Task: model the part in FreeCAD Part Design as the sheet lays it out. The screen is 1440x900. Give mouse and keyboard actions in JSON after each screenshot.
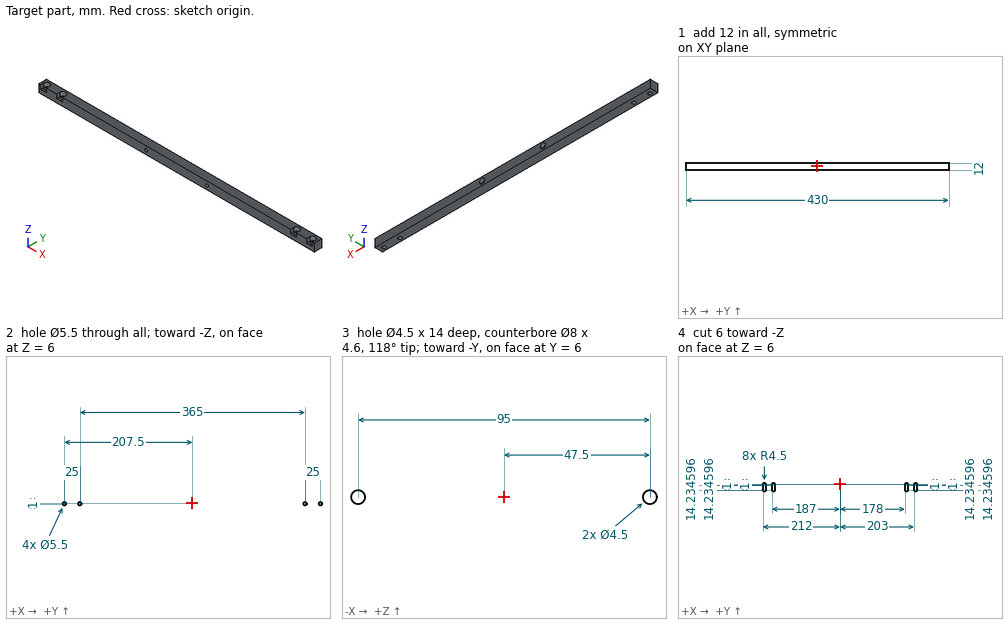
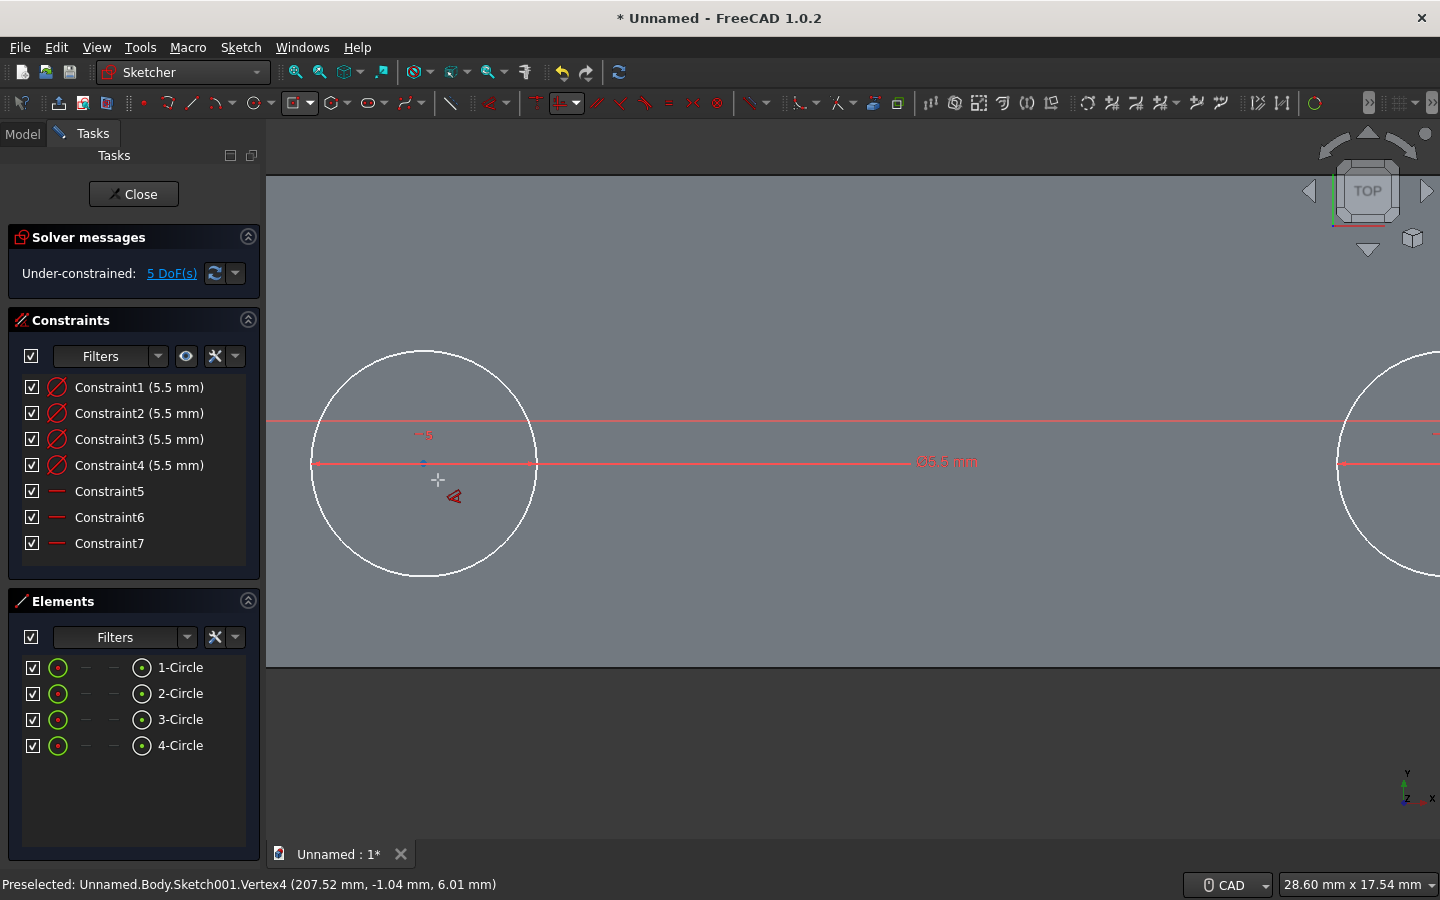
{"action": "left_click", "coordinate": [424, 464]}
{"action": "left_click", "coordinate": [390, 443]}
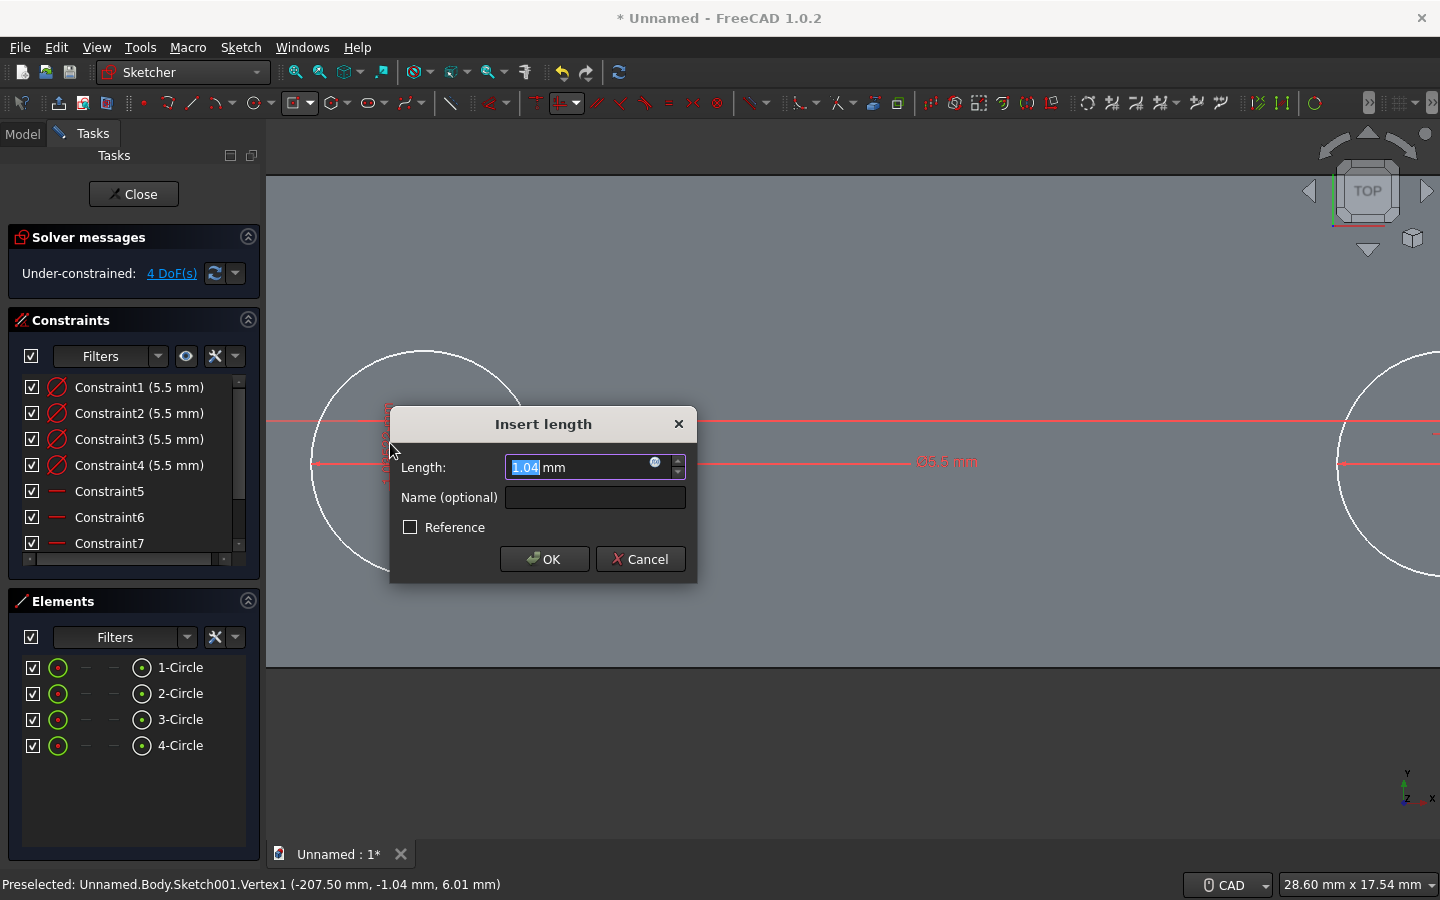
{"action": "type", "text": "1"}
{"action": "key", "text": "Return"}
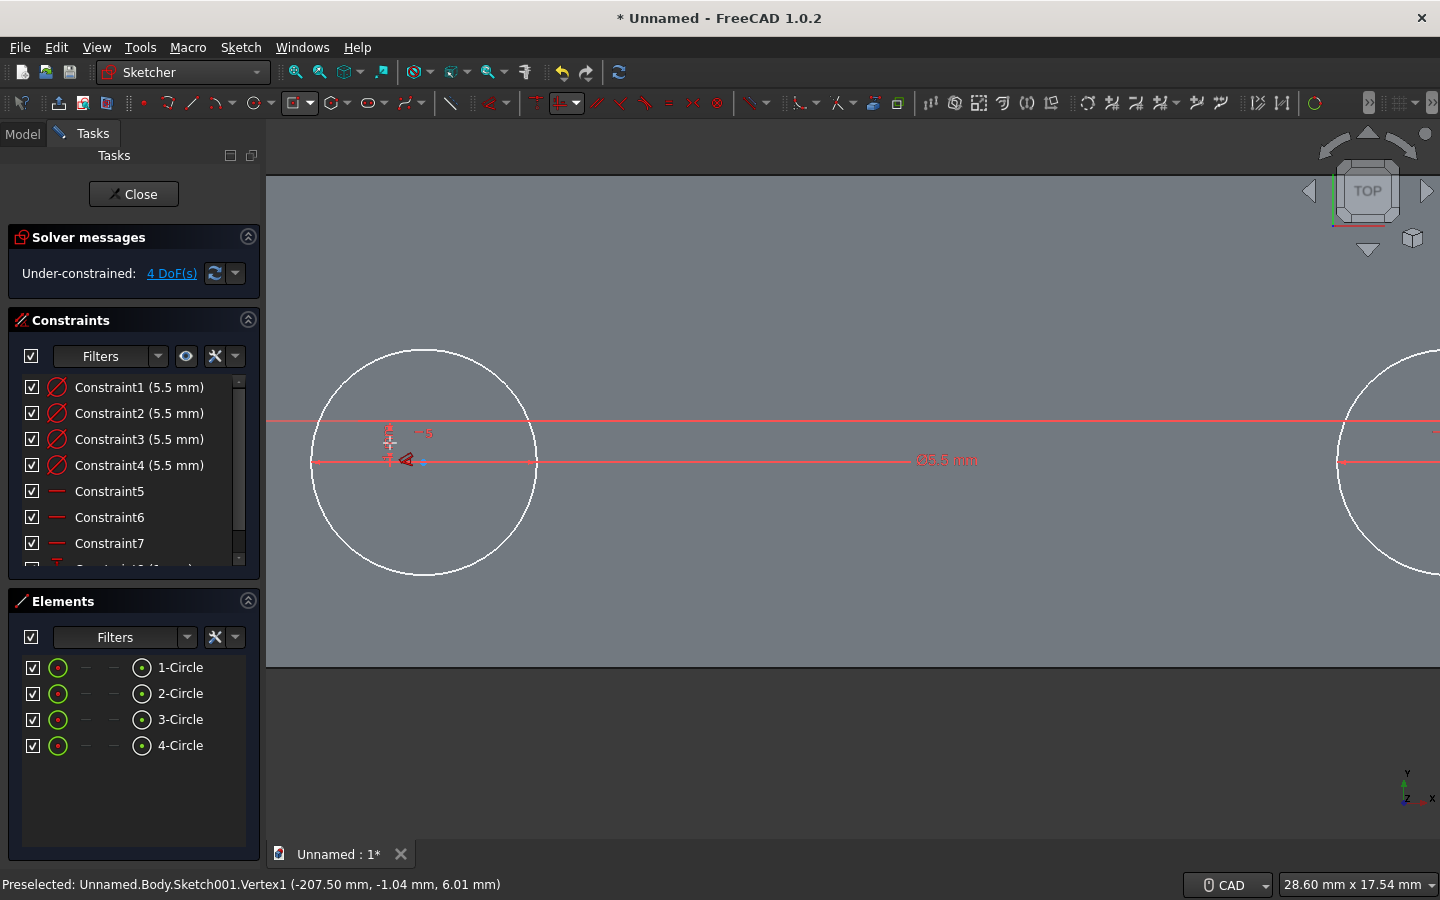
{"action": "scroll", "coordinate": [357, 480], "scroll_direction": "down", "scroll_amount": 15}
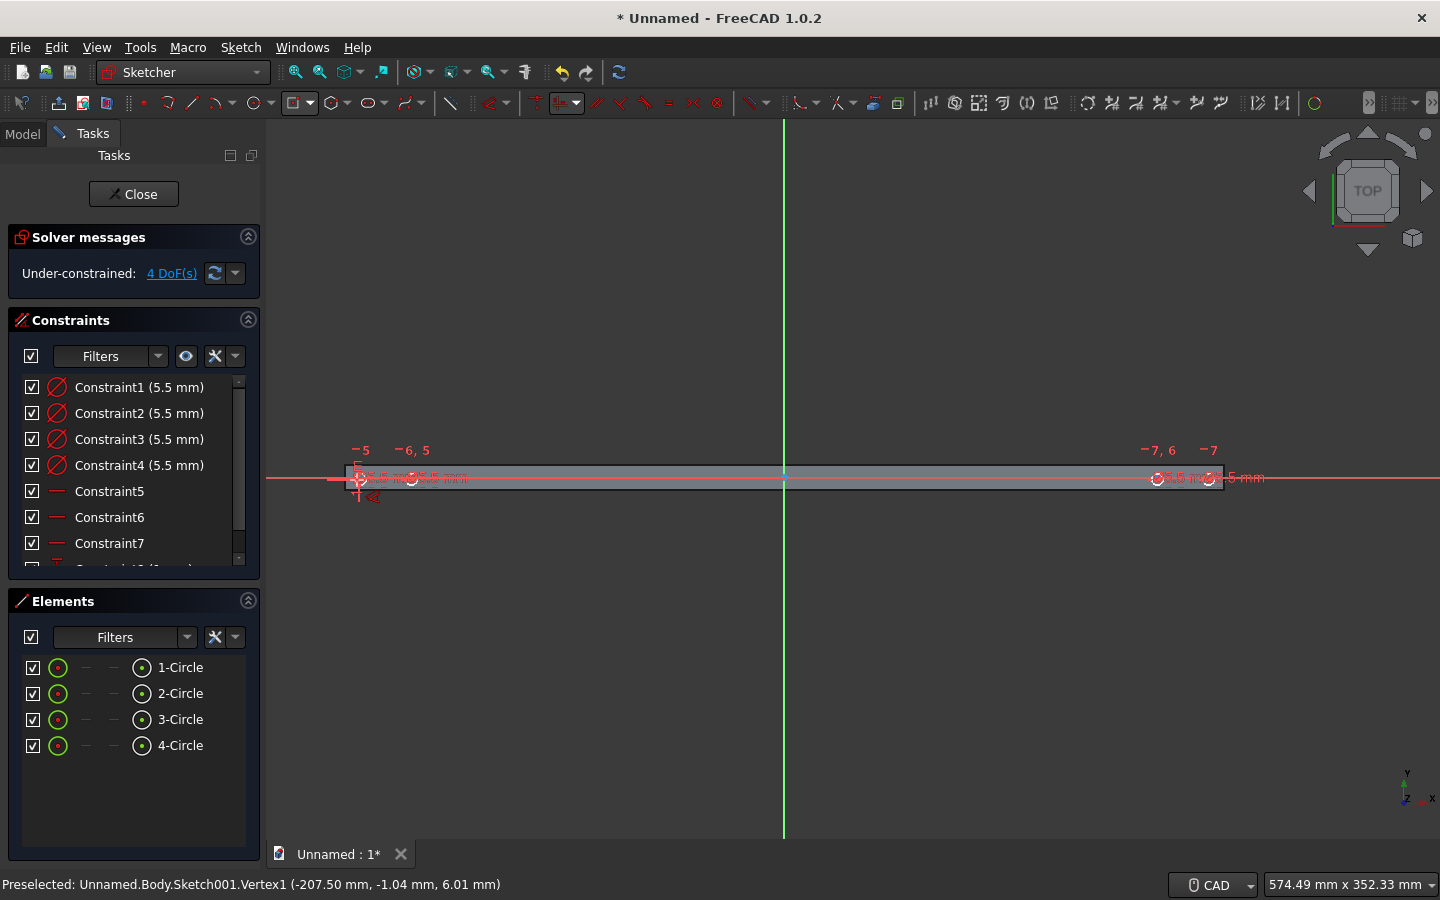
{"action": "left_click", "coordinate": [360, 480]}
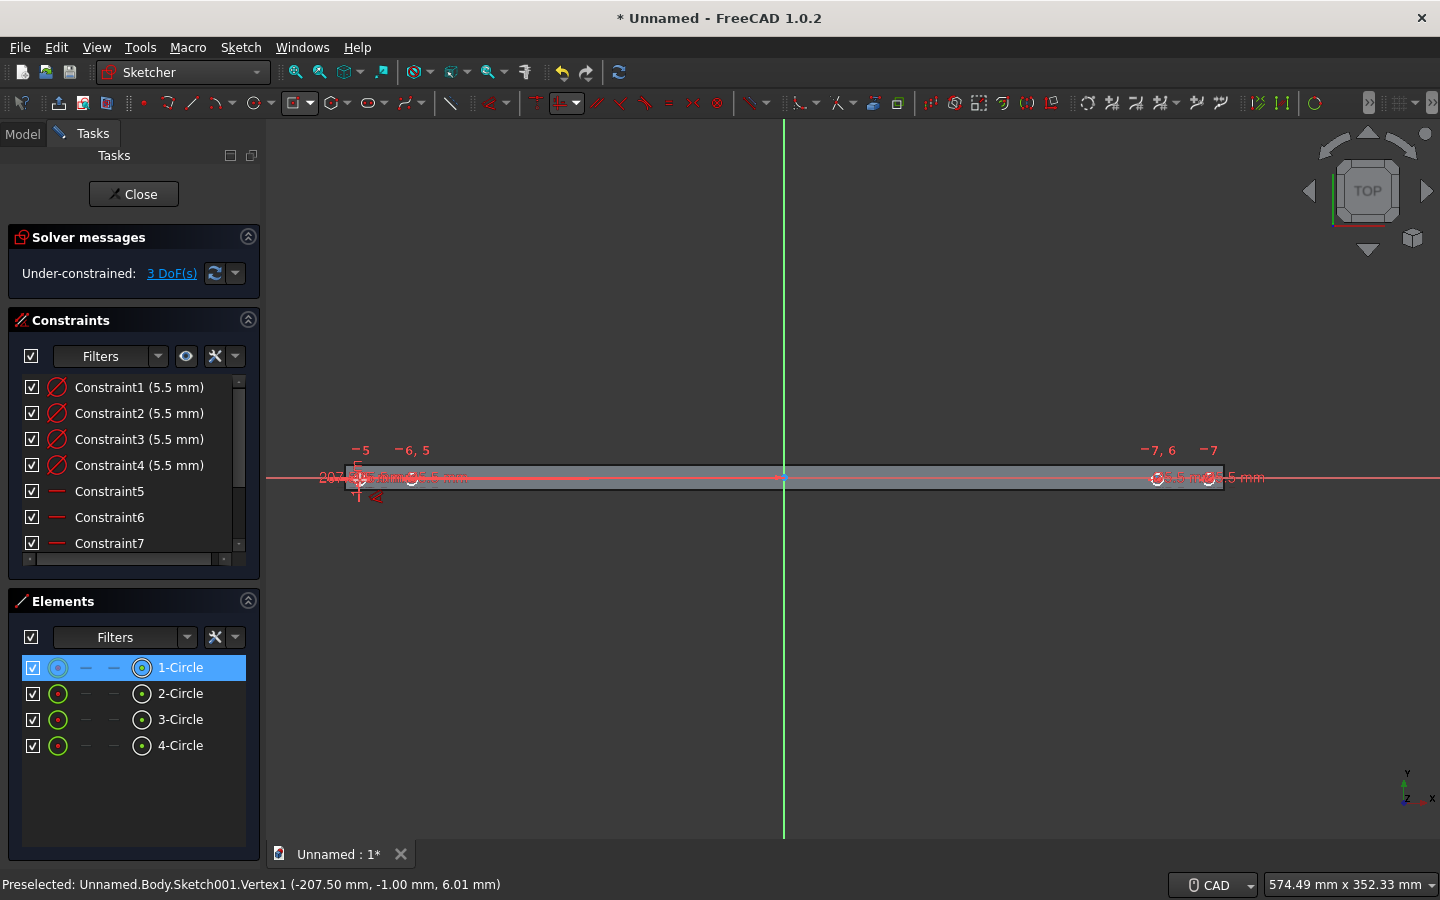
{"action": "left_click", "coordinate": [411, 480]}
{"action": "left_click", "coordinate": [386, 514]}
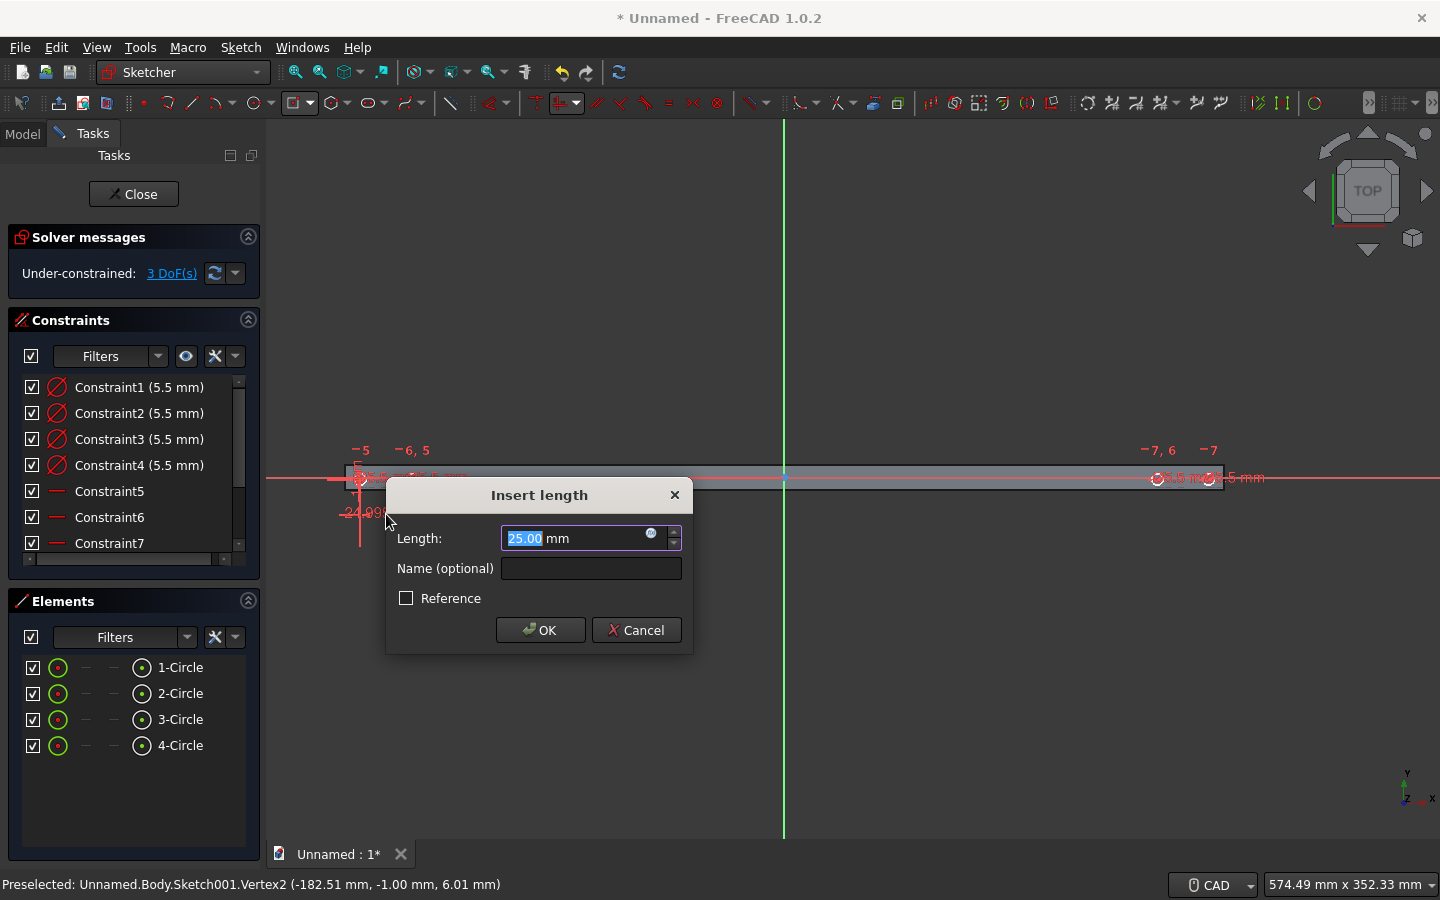
{"action": "type", "text": "25"}
{"action": "key", "text": "Return"}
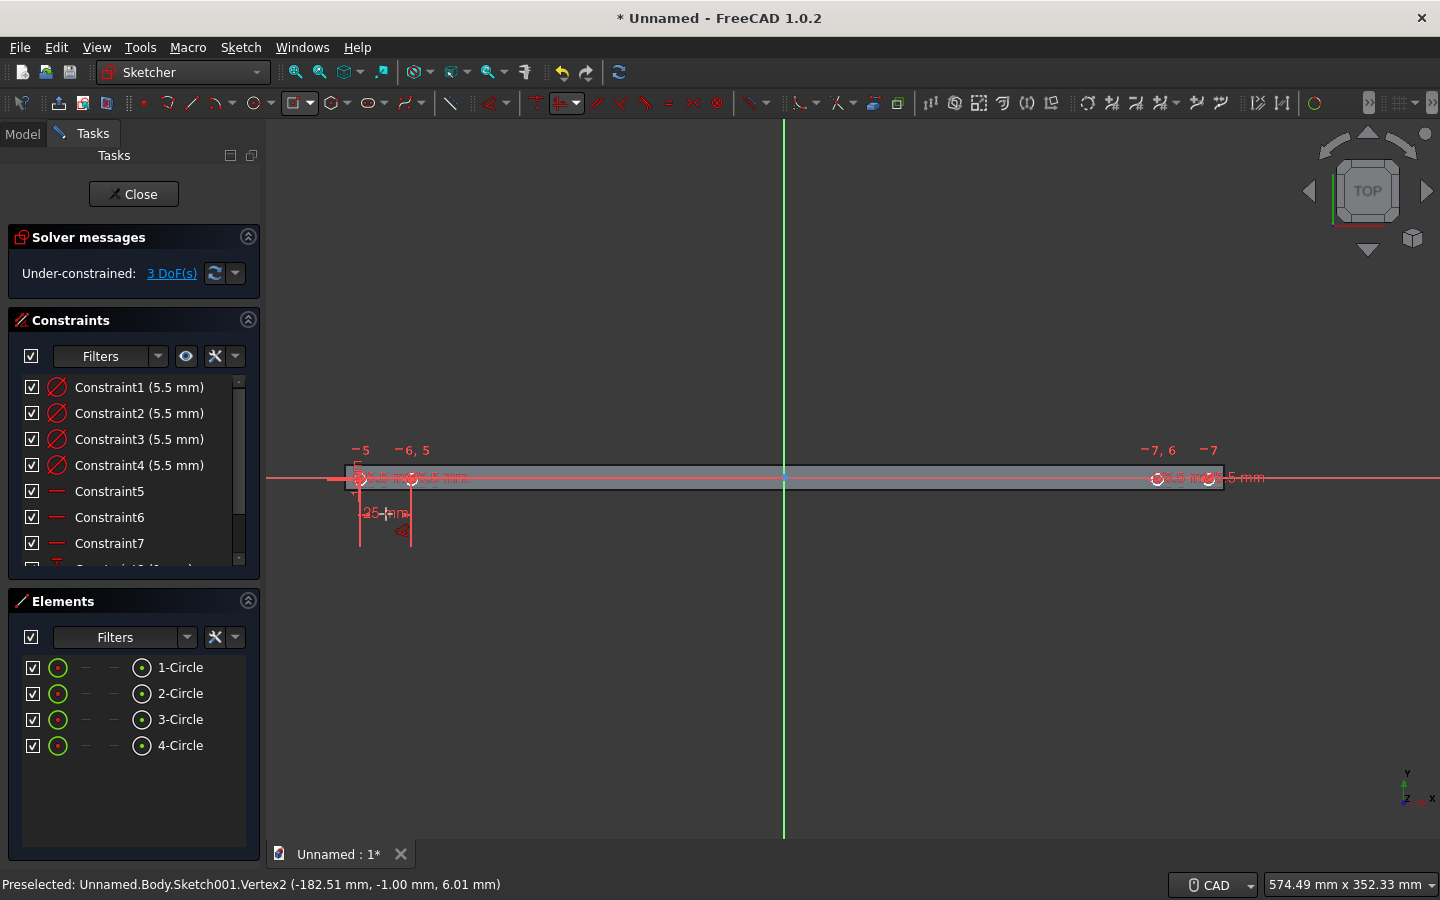
{"action": "left_click", "coordinate": [1157, 480]}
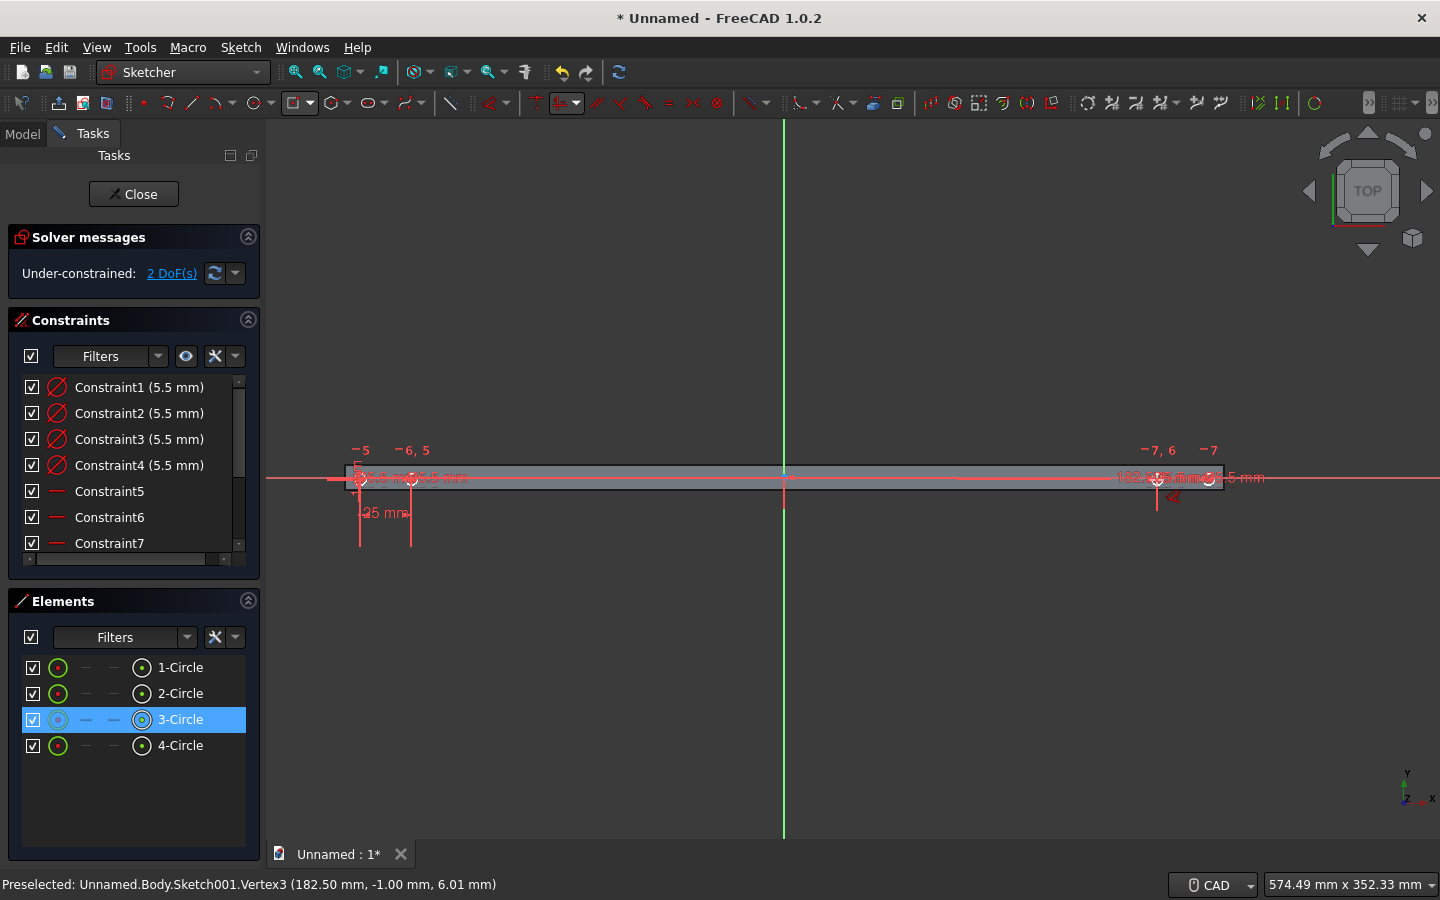
{"action": "left_click", "coordinate": [1209, 480]}
{"action": "left_click", "coordinate": [1183, 514]}